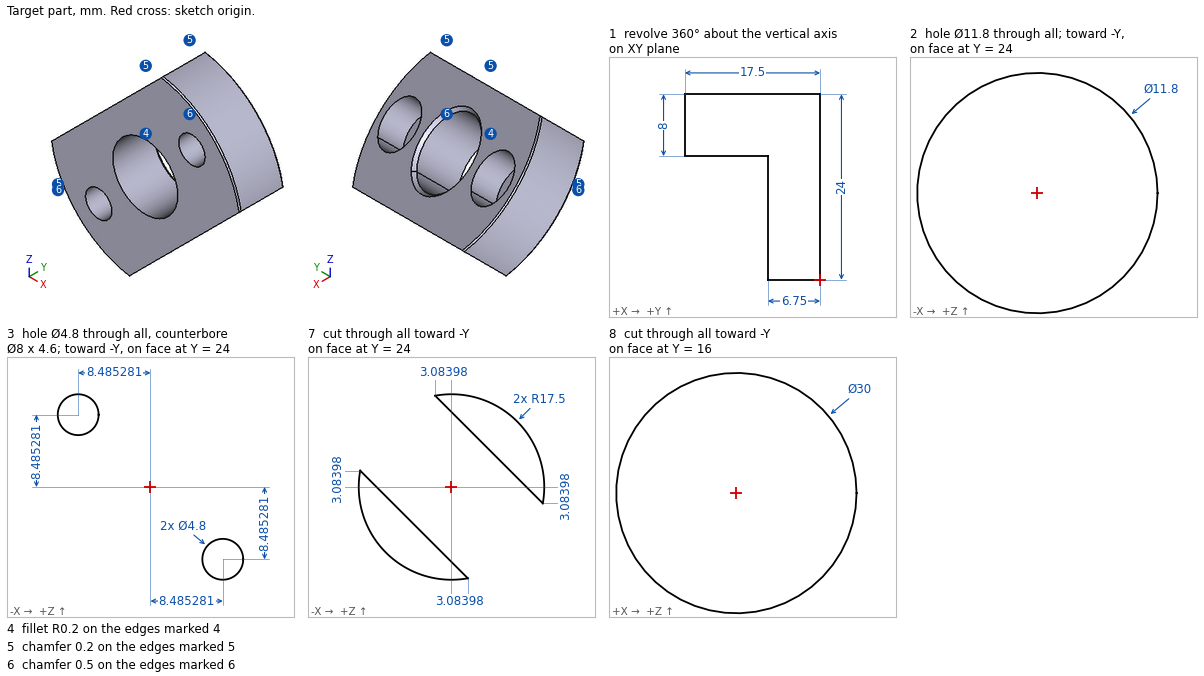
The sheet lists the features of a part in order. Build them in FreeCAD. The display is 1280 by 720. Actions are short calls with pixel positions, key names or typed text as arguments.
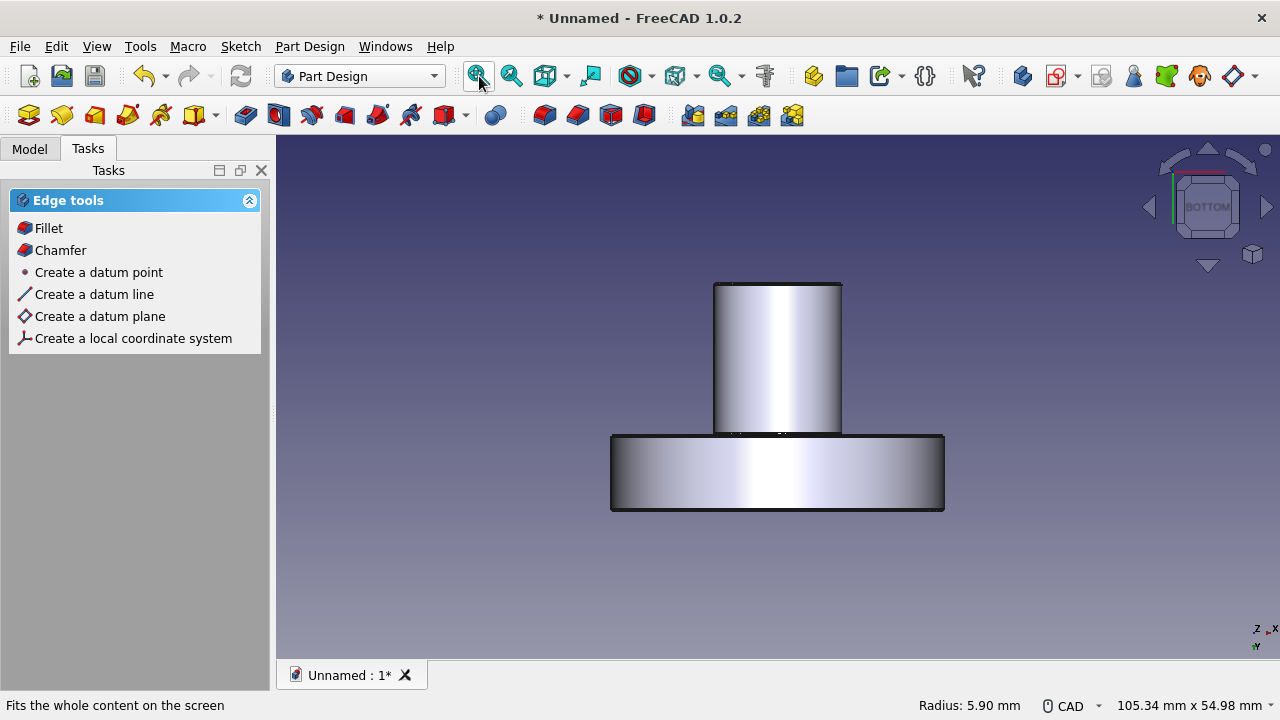
key(4)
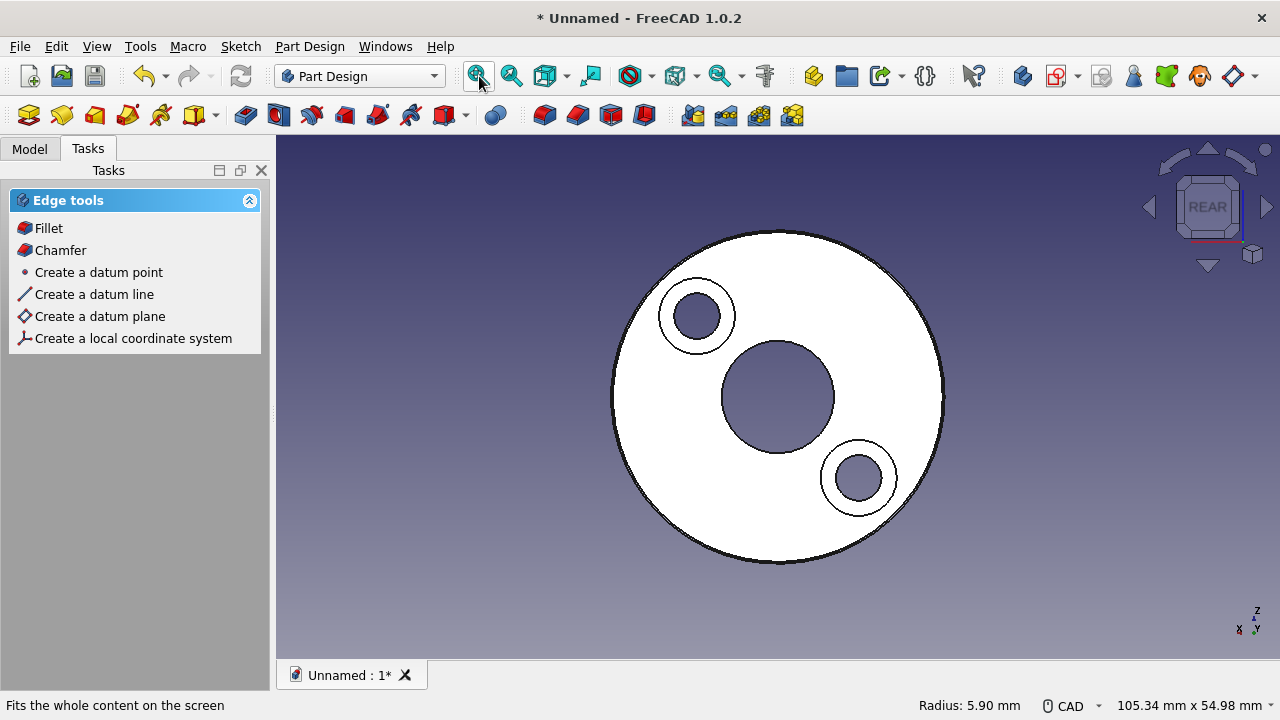
click(834, 396, ctrl)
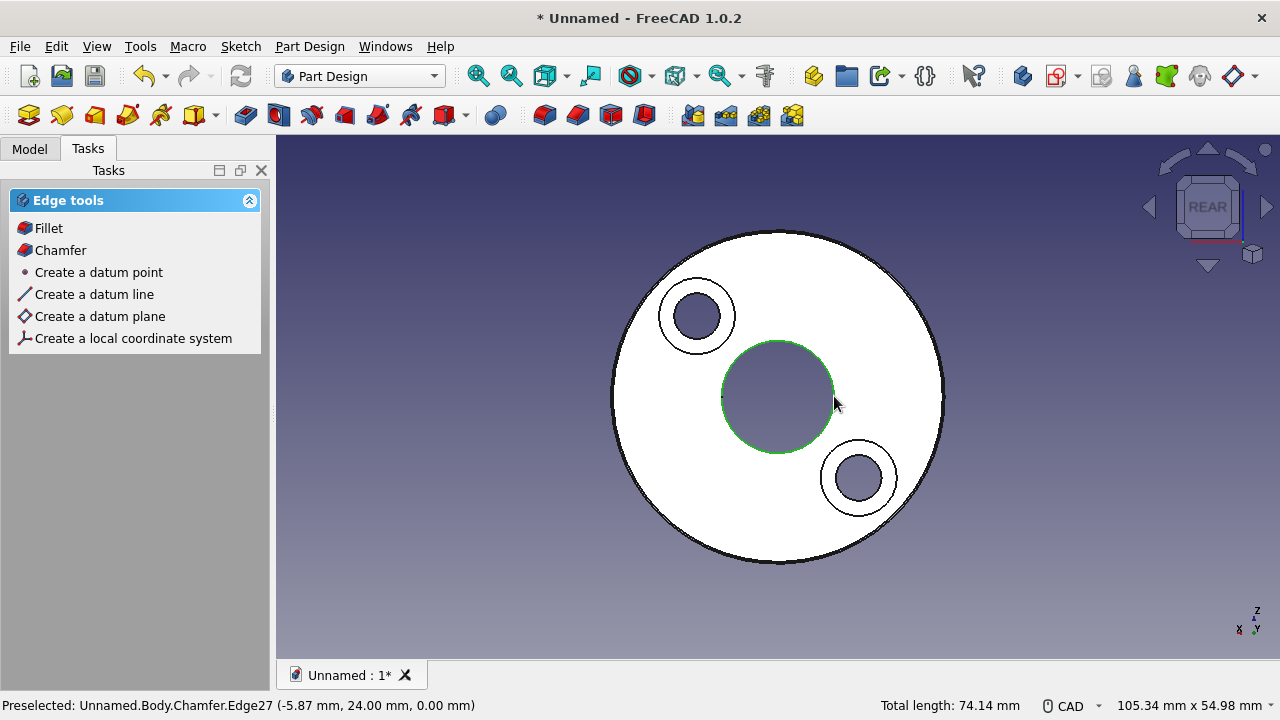
click(578, 116)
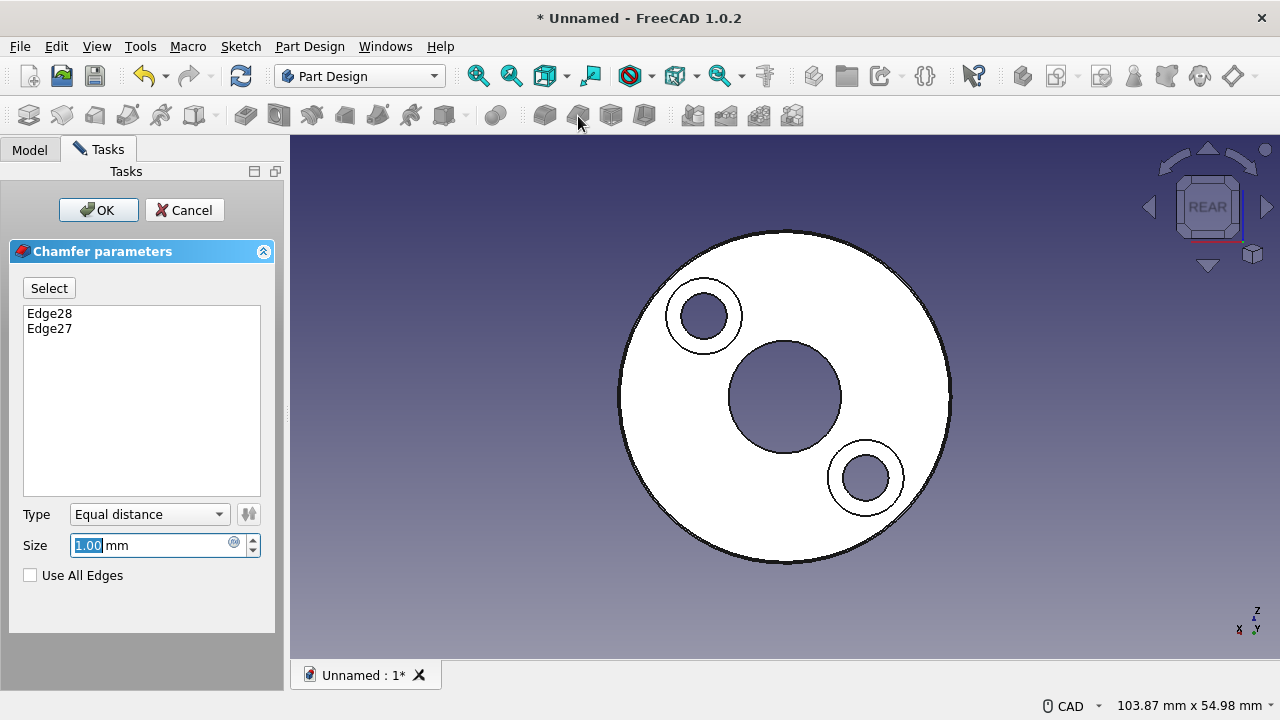
text(0.5)
key(Tab)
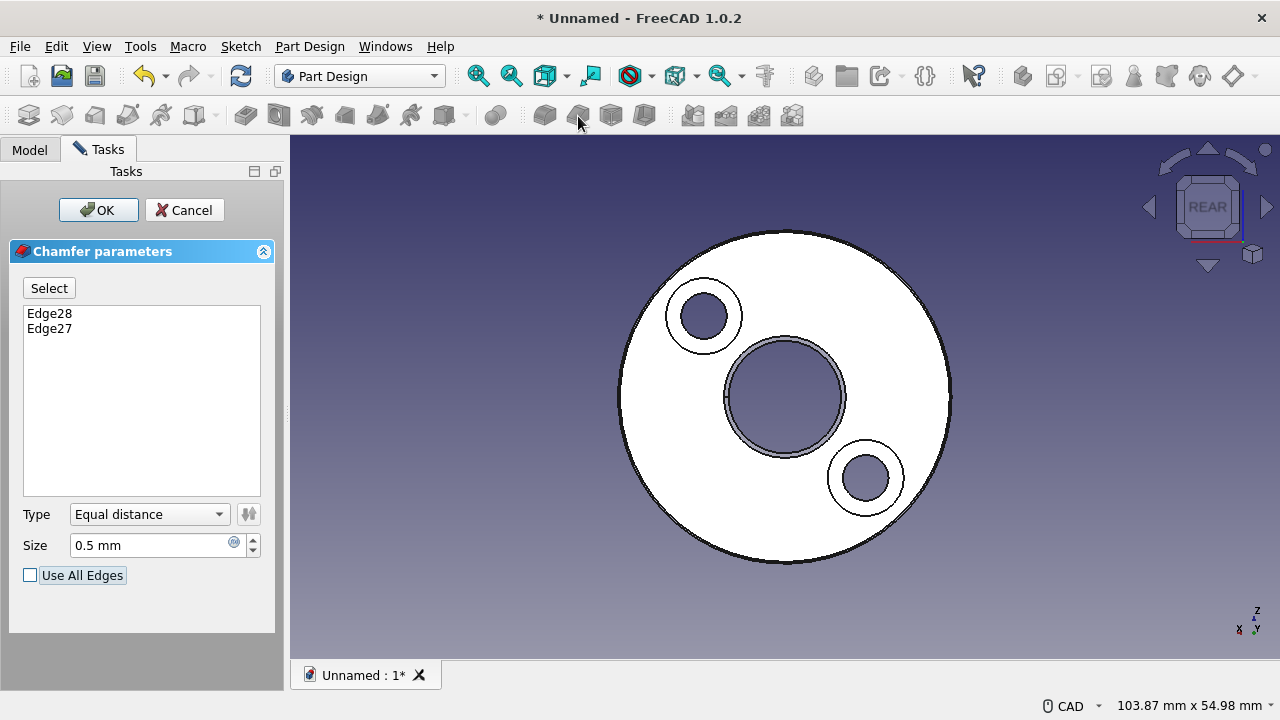
click(99, 210)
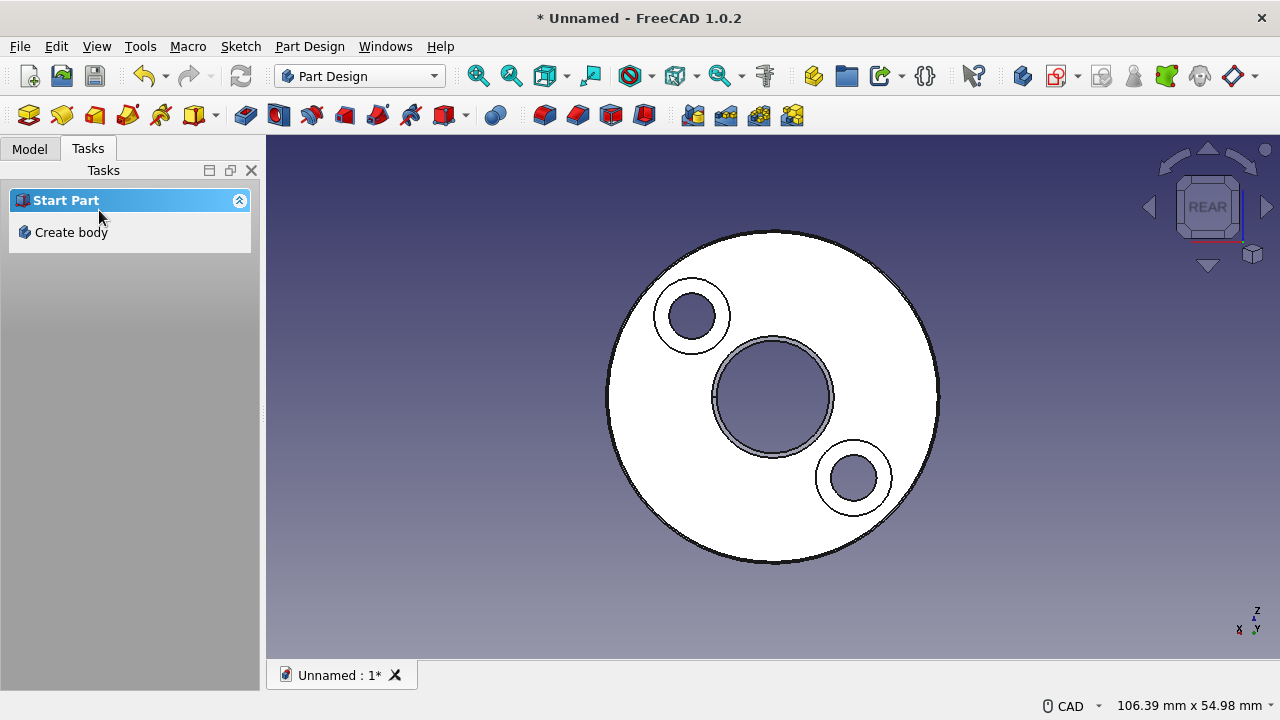
click(679, 443)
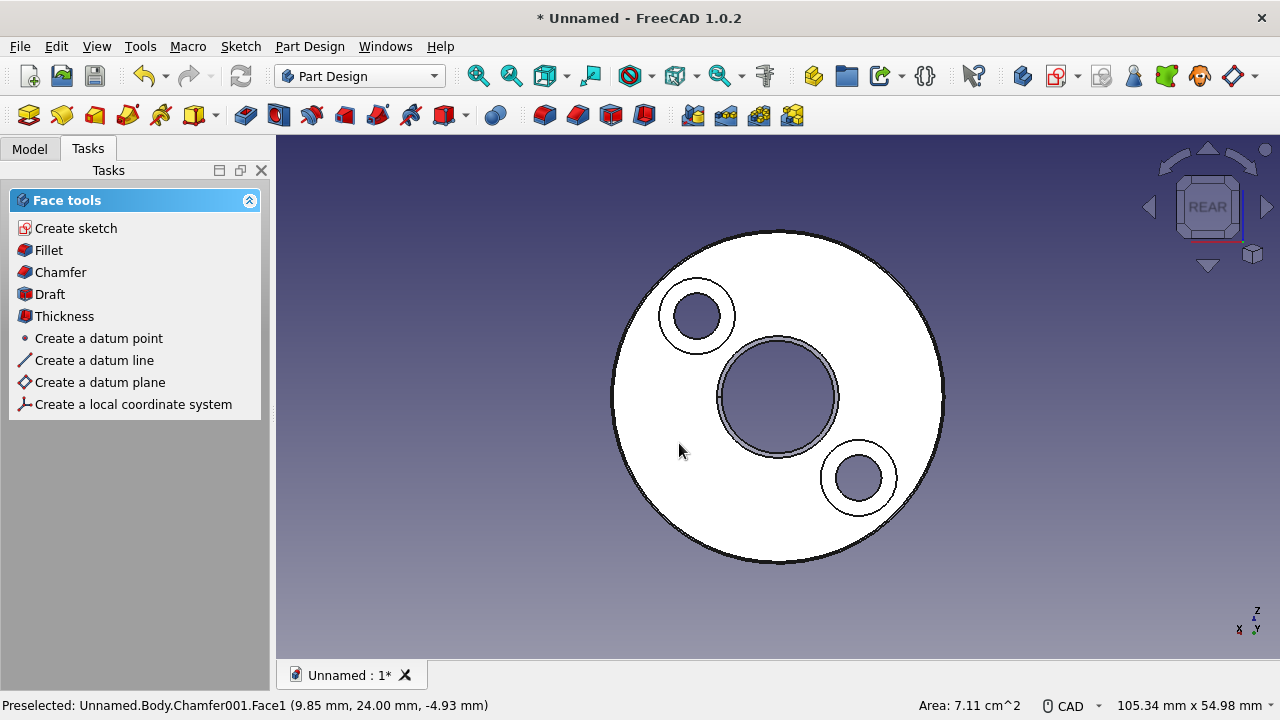
click(1056, 76)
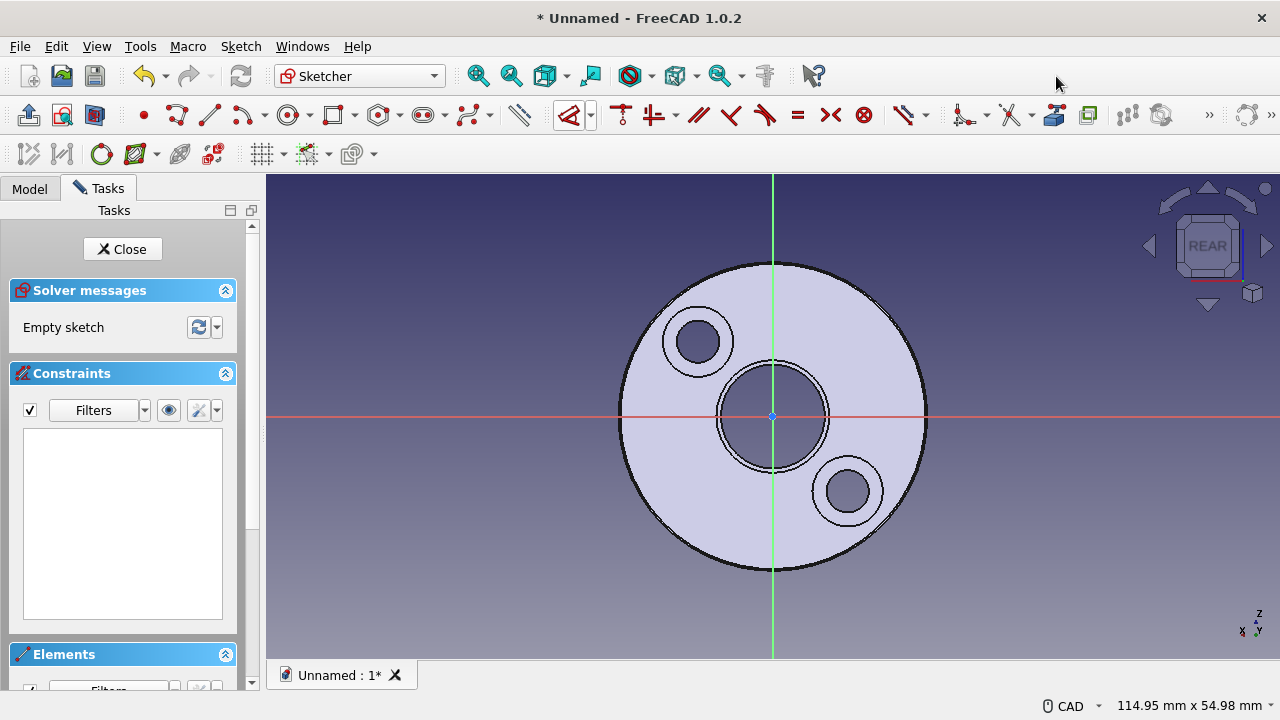
click(210, 116)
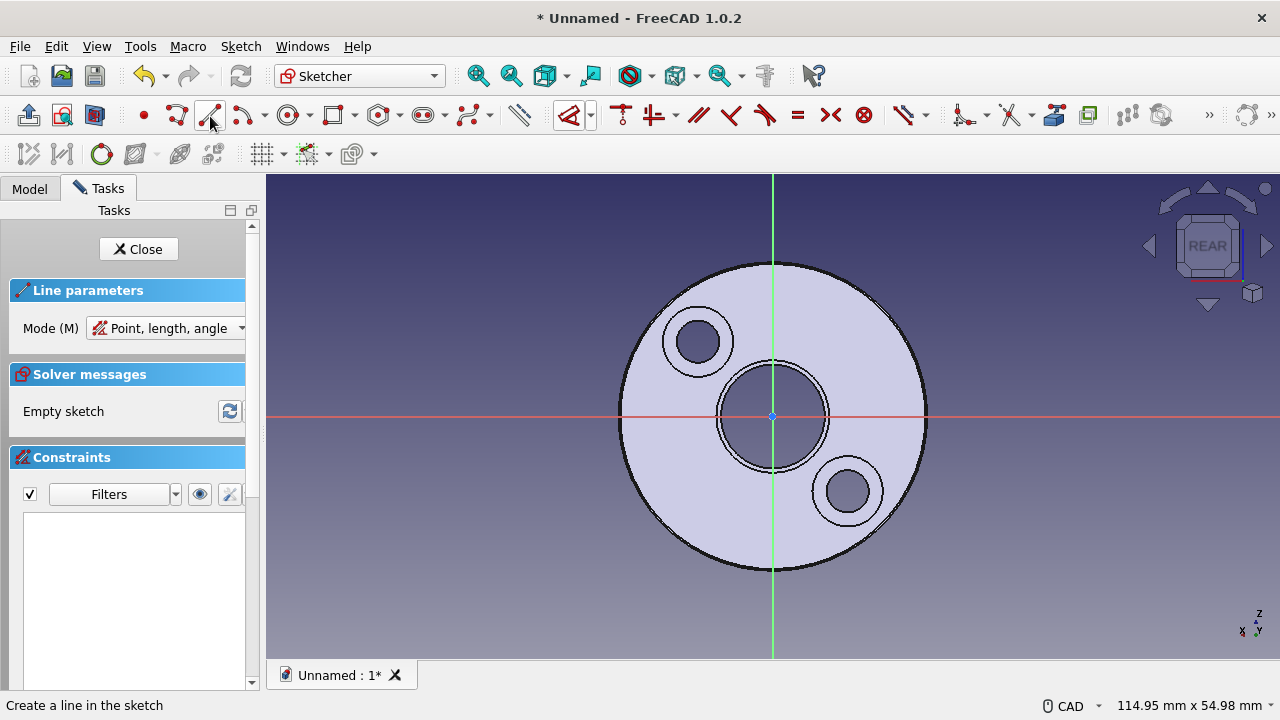
click(746, 265)
click(925, 444)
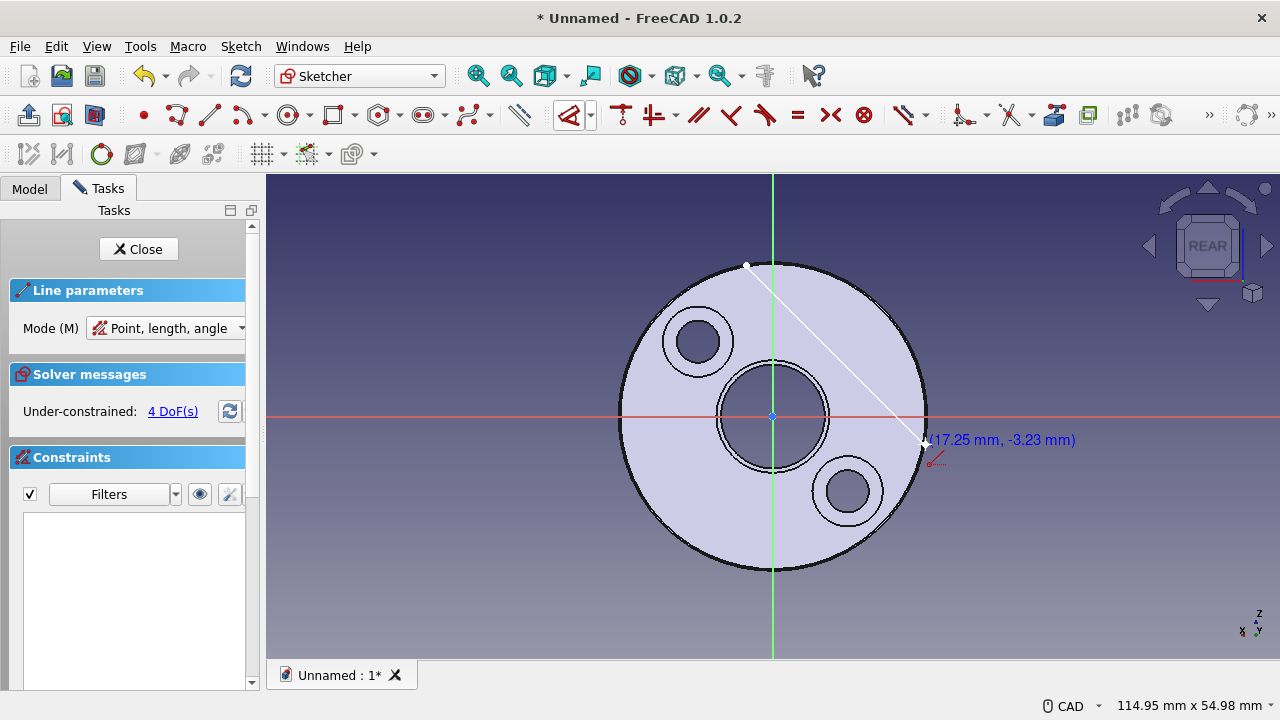
key(g)
key(3)
key(a)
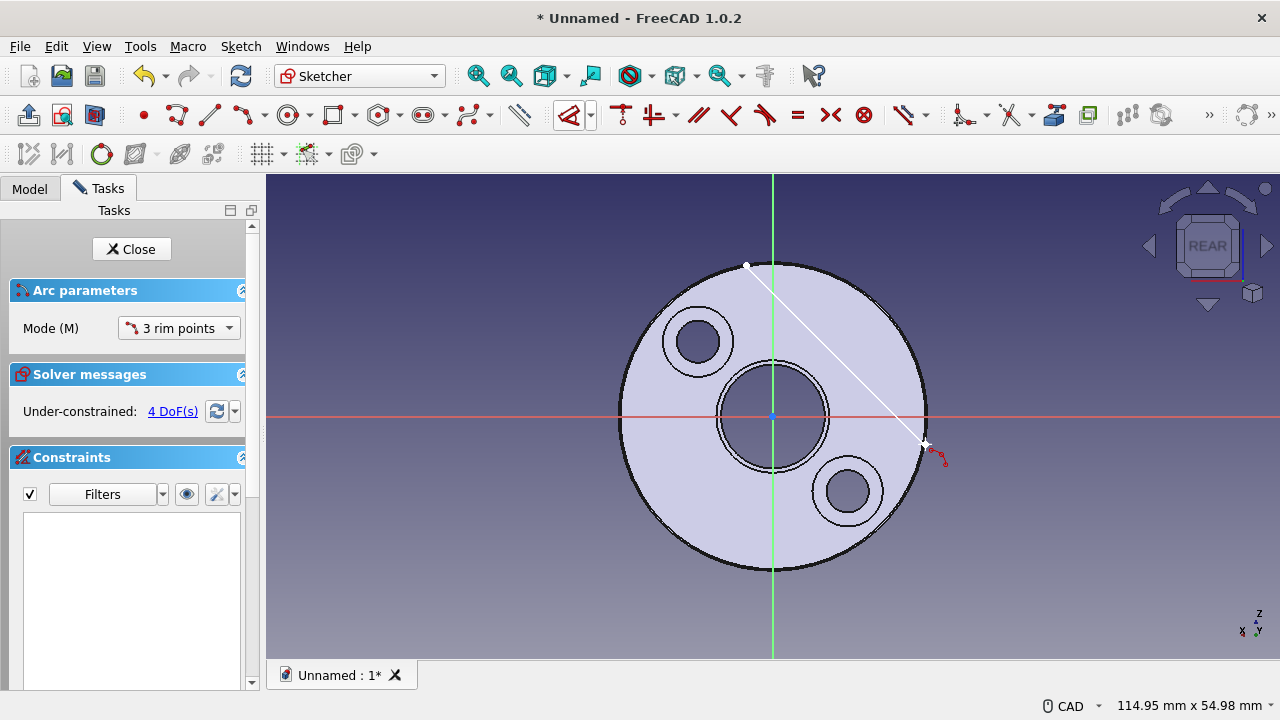
click(925, 445)
click(746, 266)
click(882, 307)